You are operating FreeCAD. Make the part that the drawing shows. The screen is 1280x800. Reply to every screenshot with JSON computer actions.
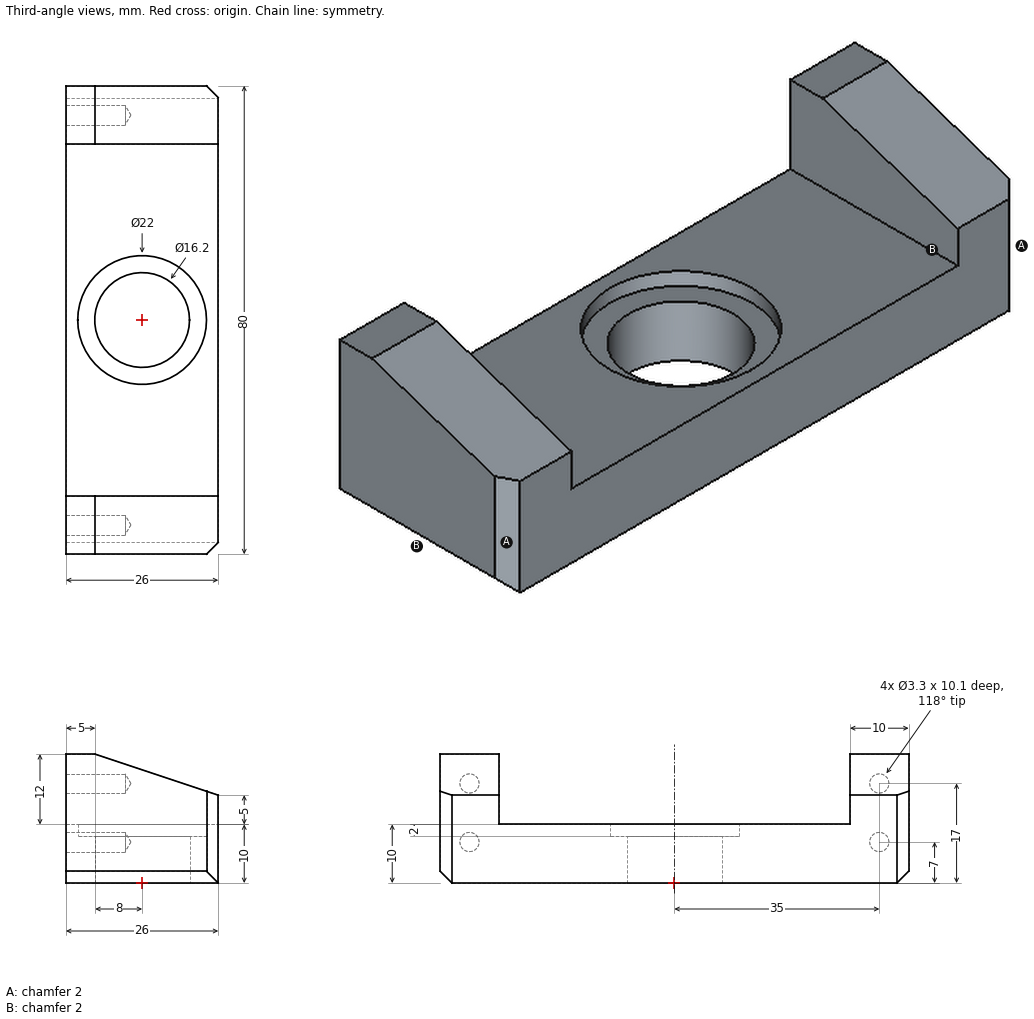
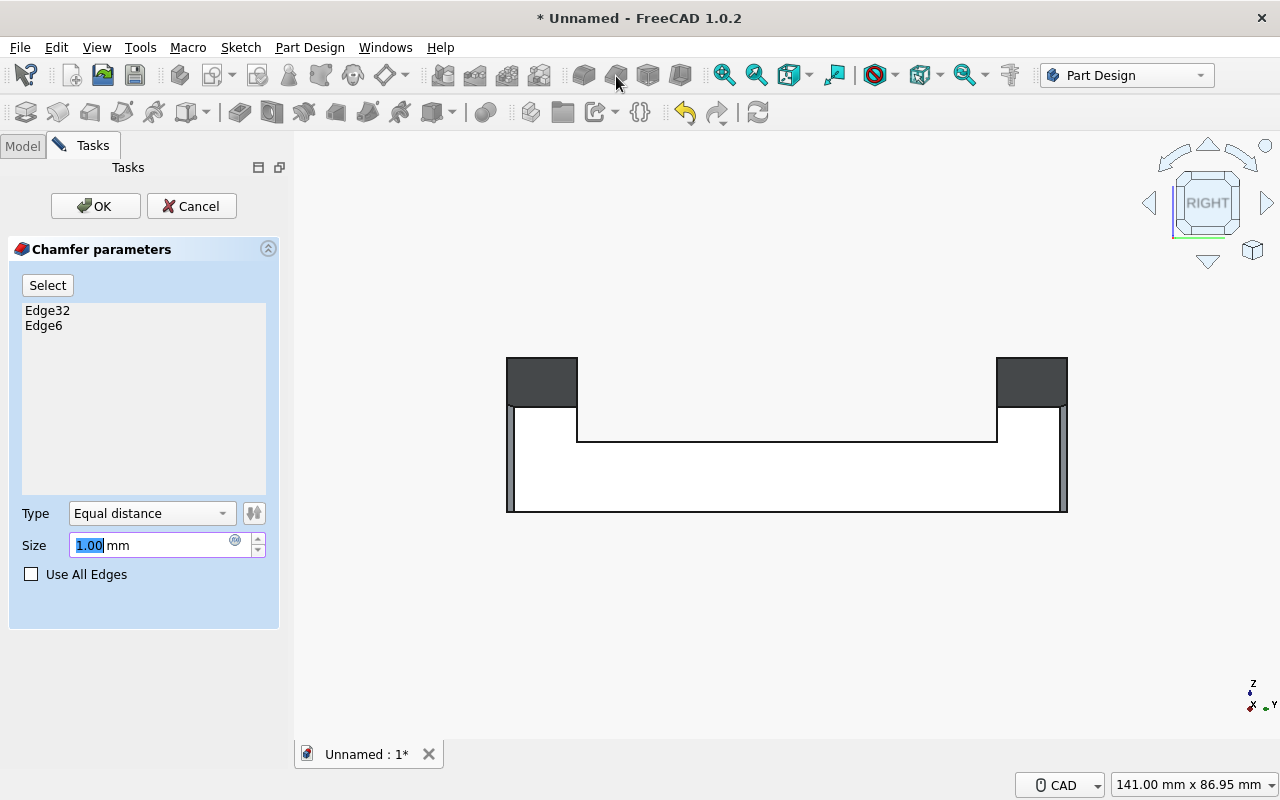
{"action": "type", "text": "2"}
{"action": "key", "text": "Tab"}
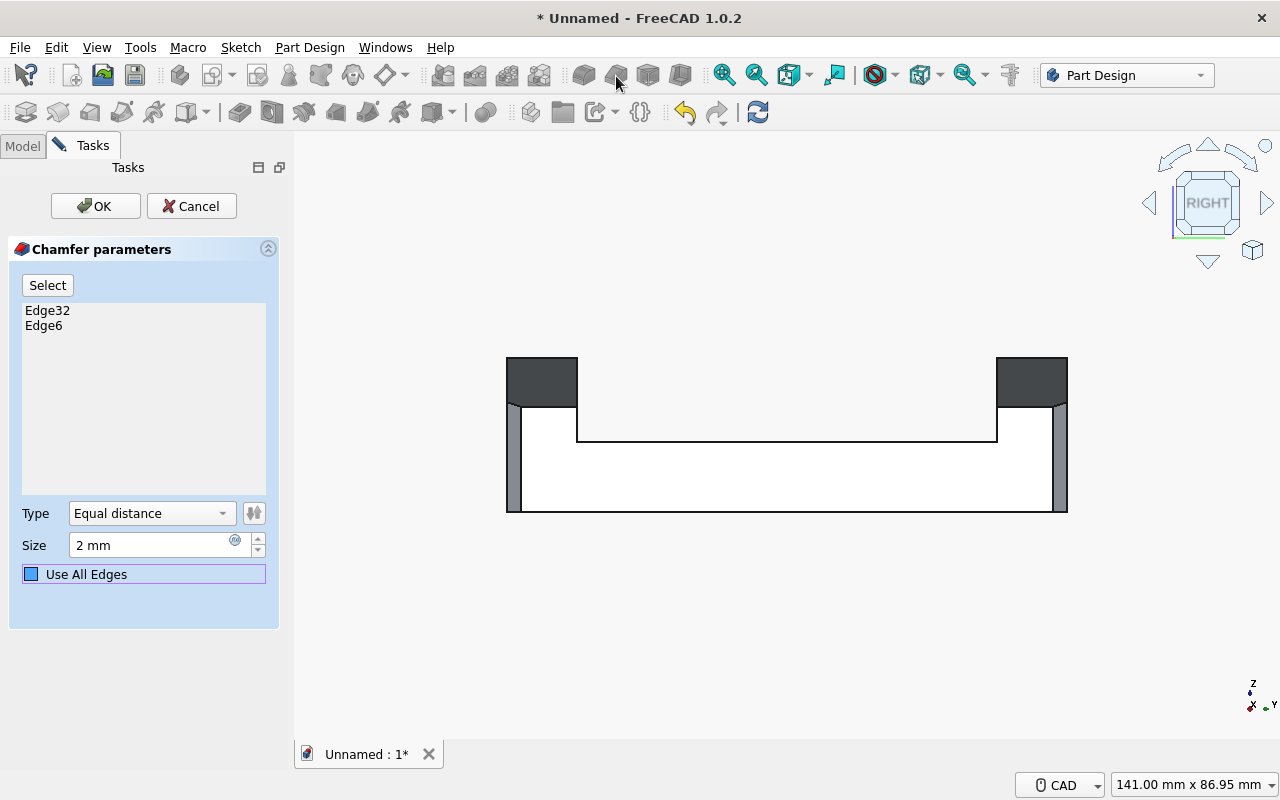
{"action": "left_click", "coordinate": [96, 206]}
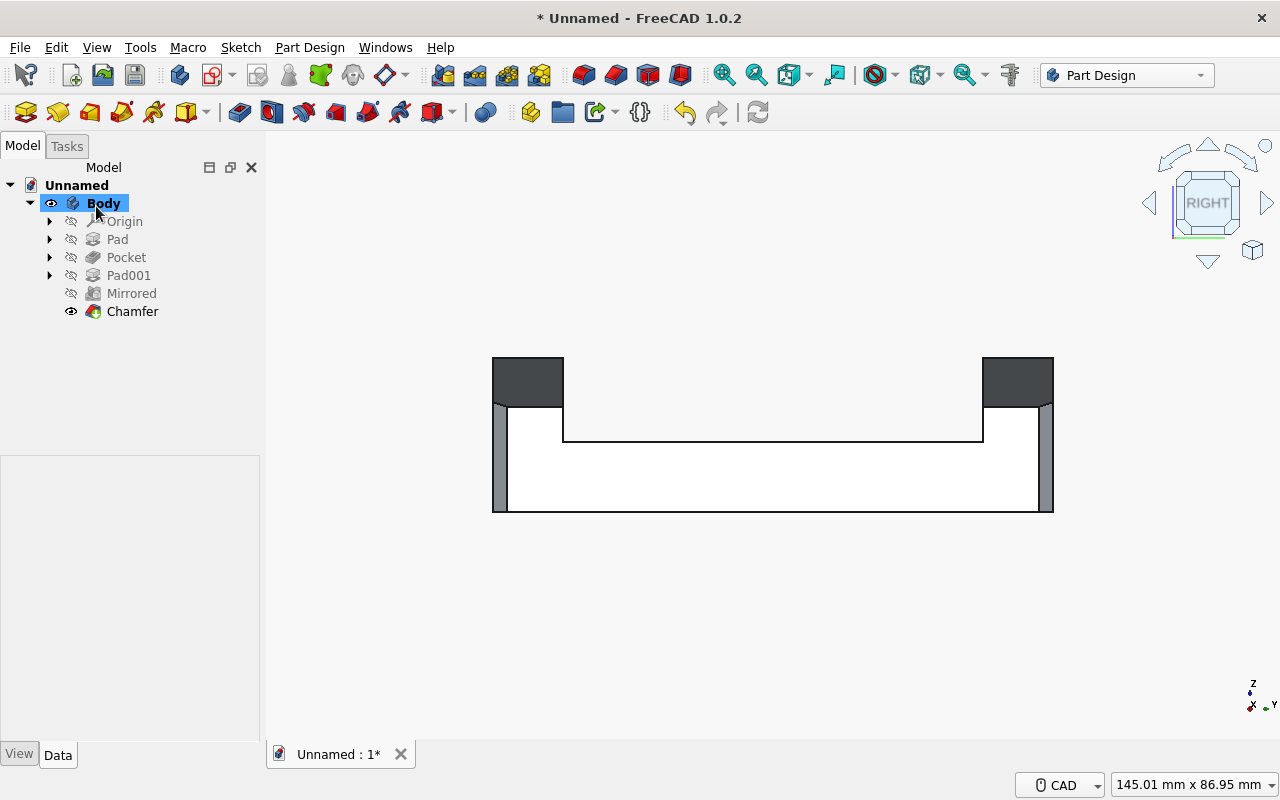
{"action": "key", "text": "0"}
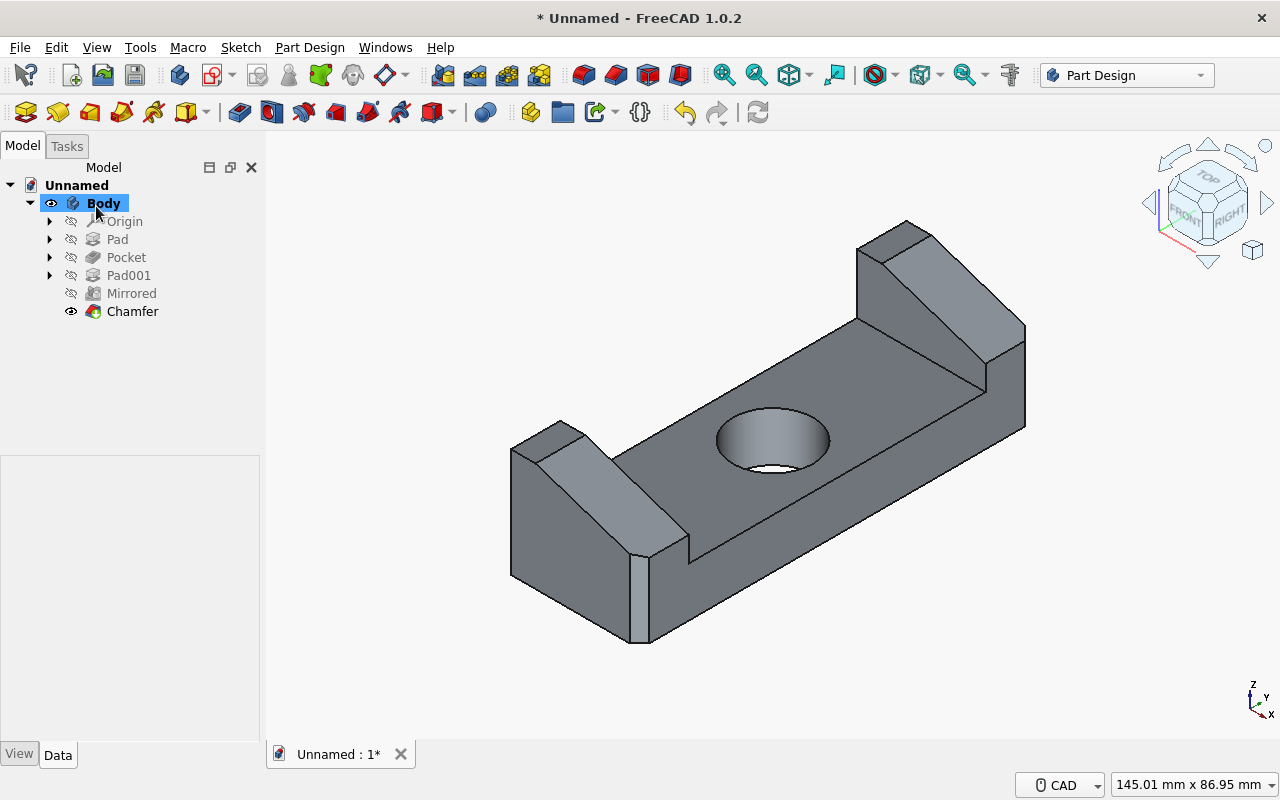
{"action": "key", "text": "2"}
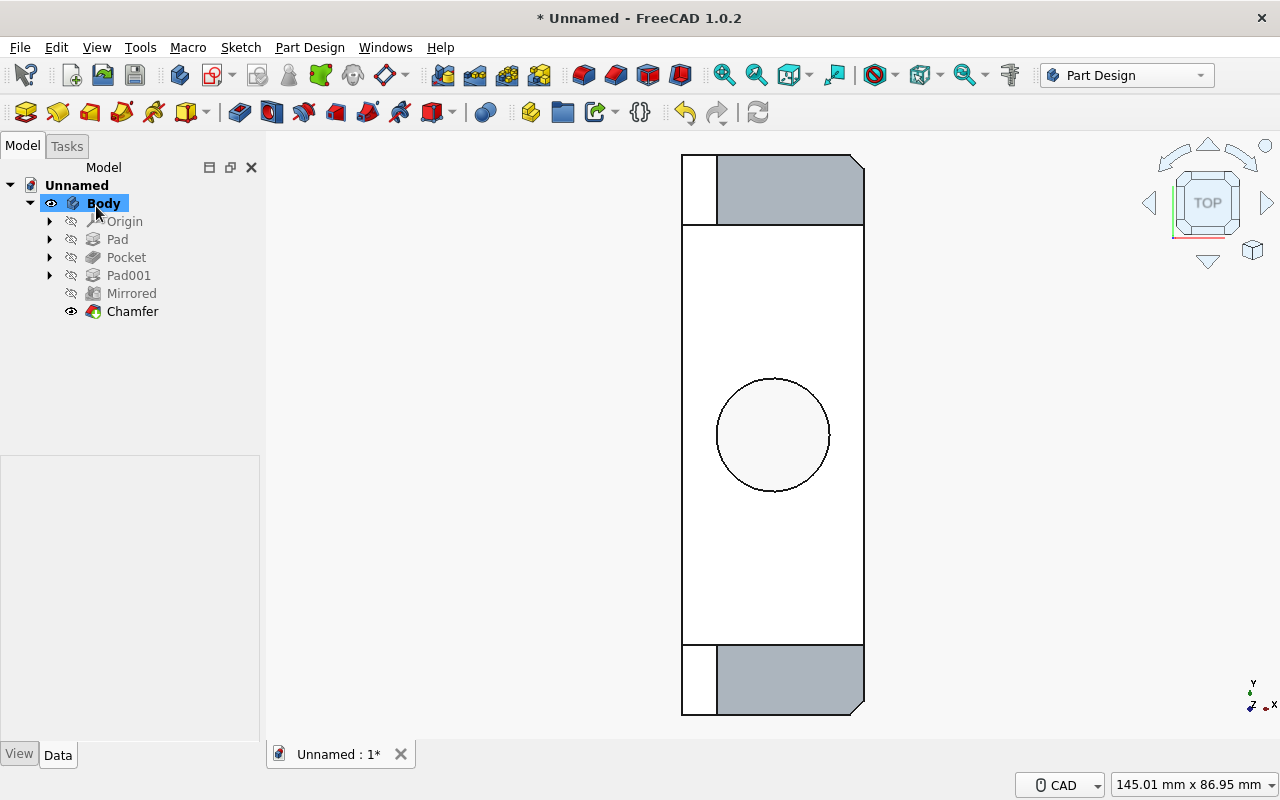
{"action": "key", "text": "1"}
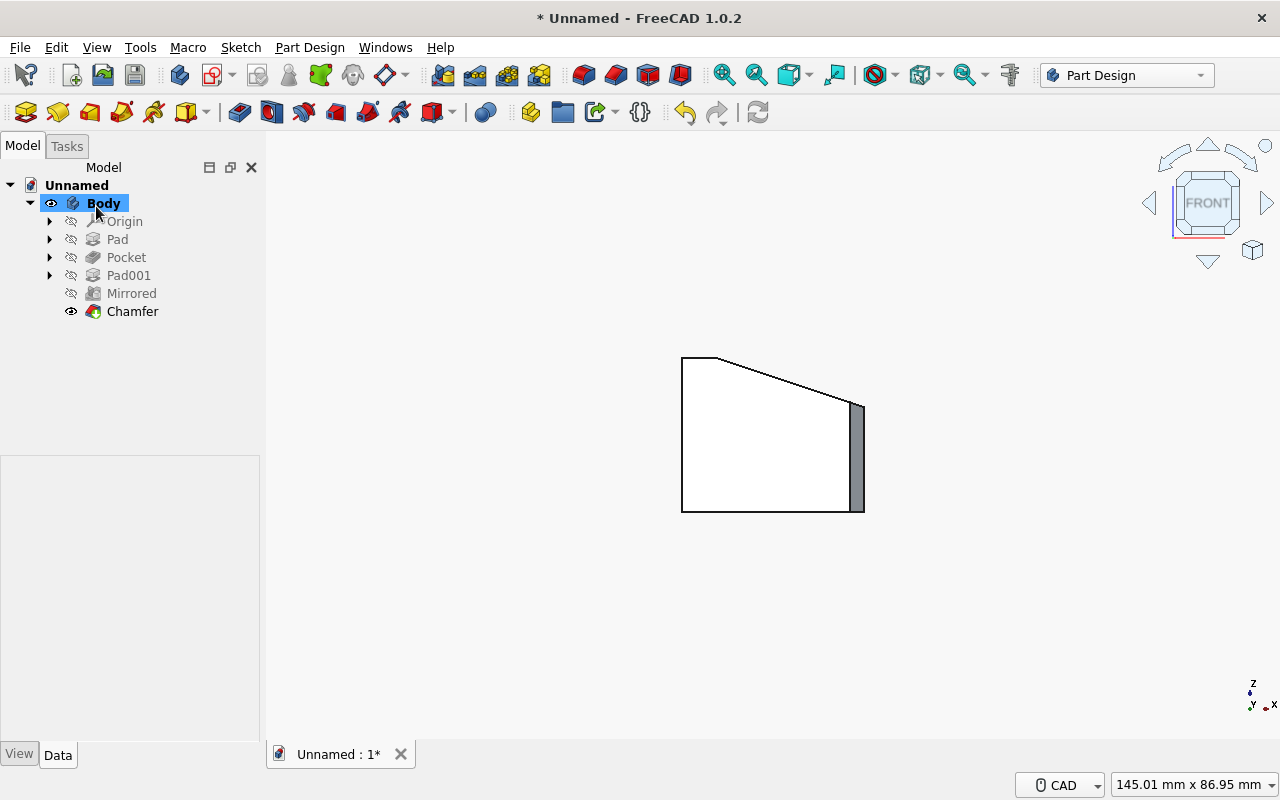
{"action": "left_click", "coordinate": [726, 76]}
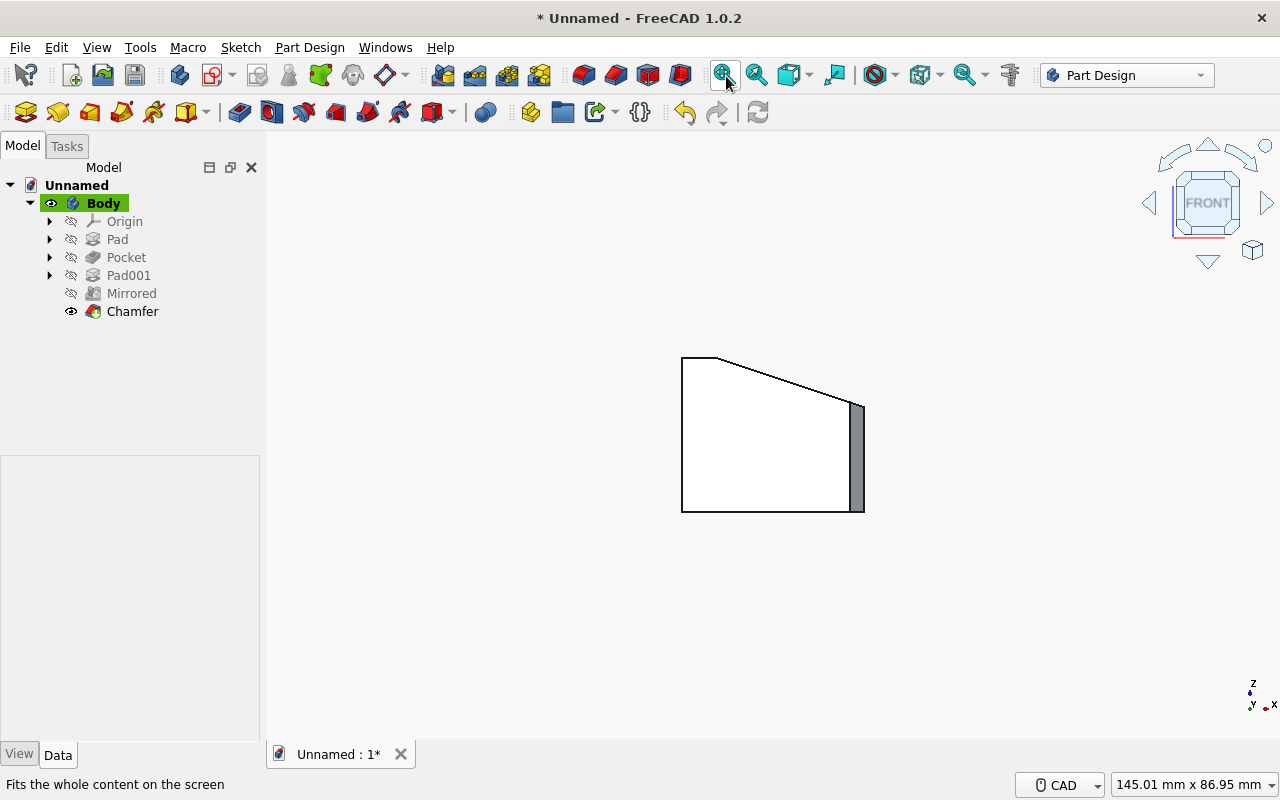
{"action": "left_click", "coordinate": [766, 511]}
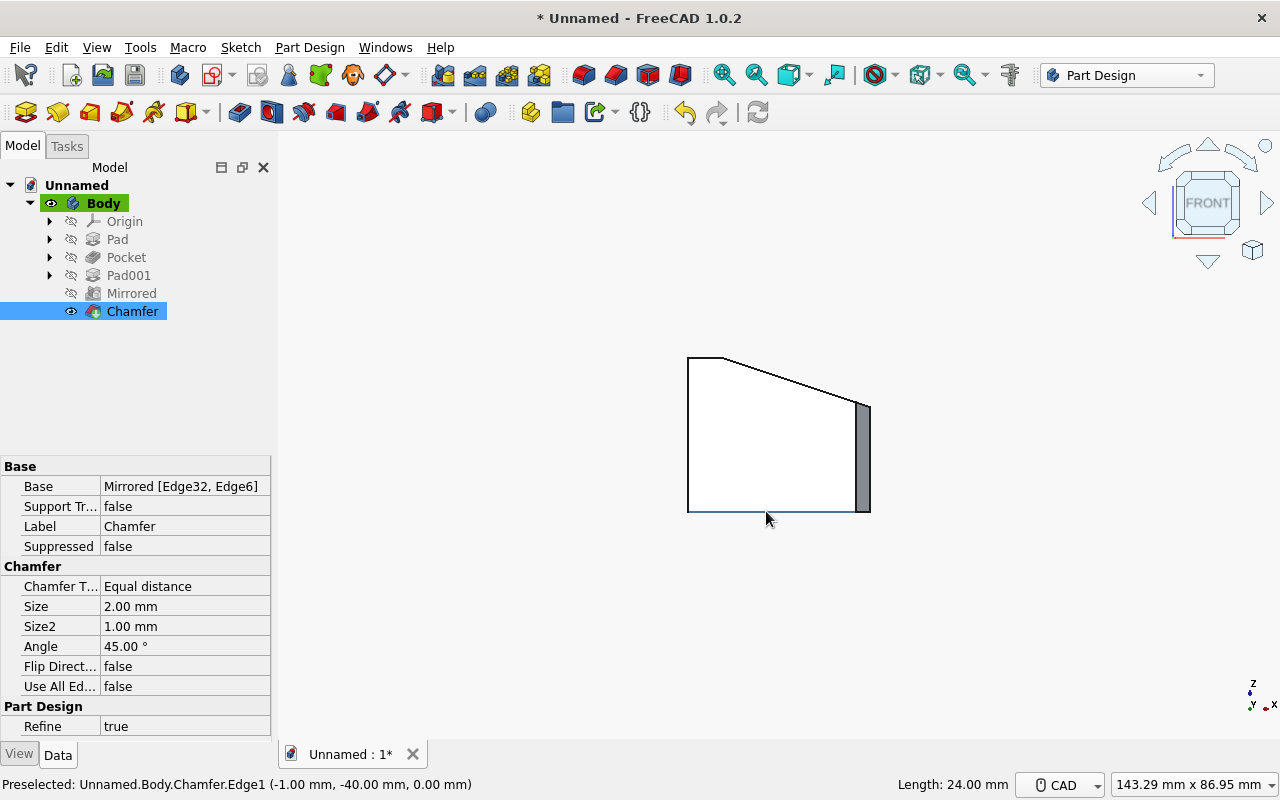
{"action": "key", "text": "3"}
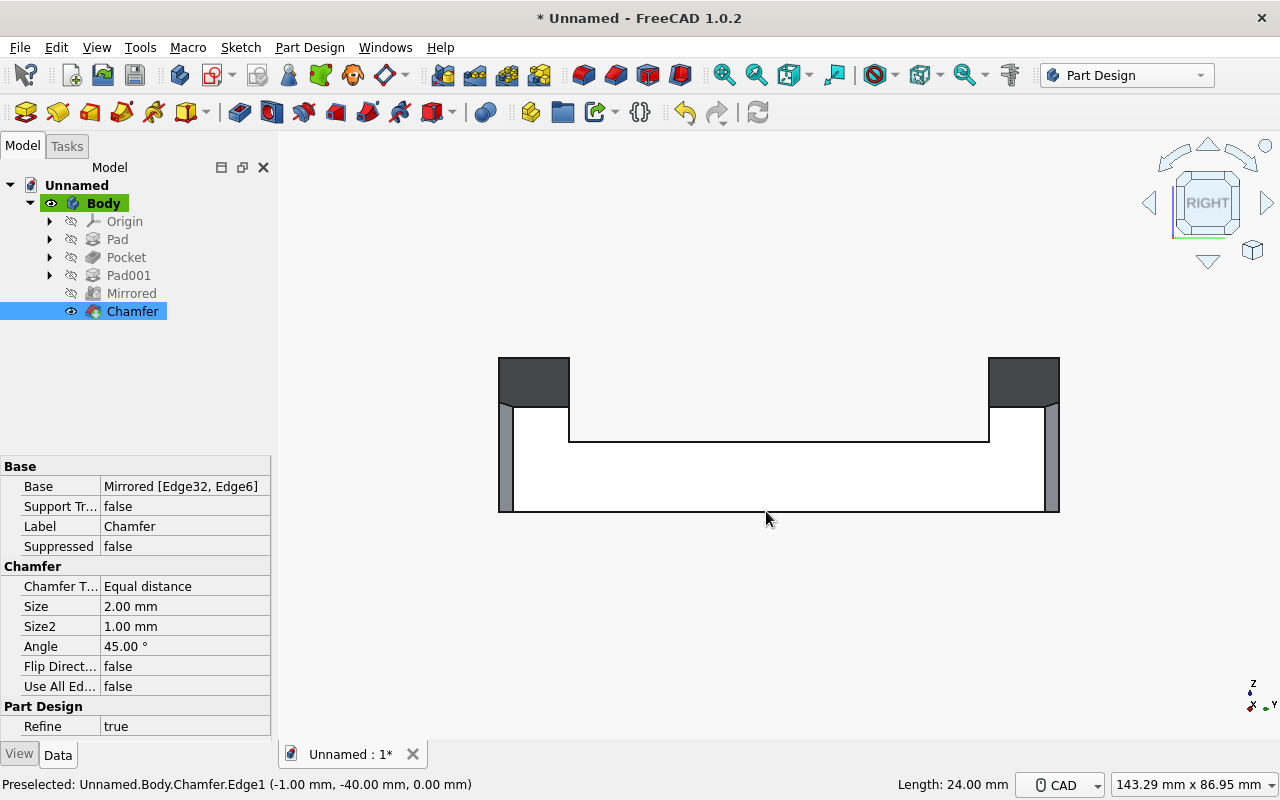
{"action": "key", "text": "5"}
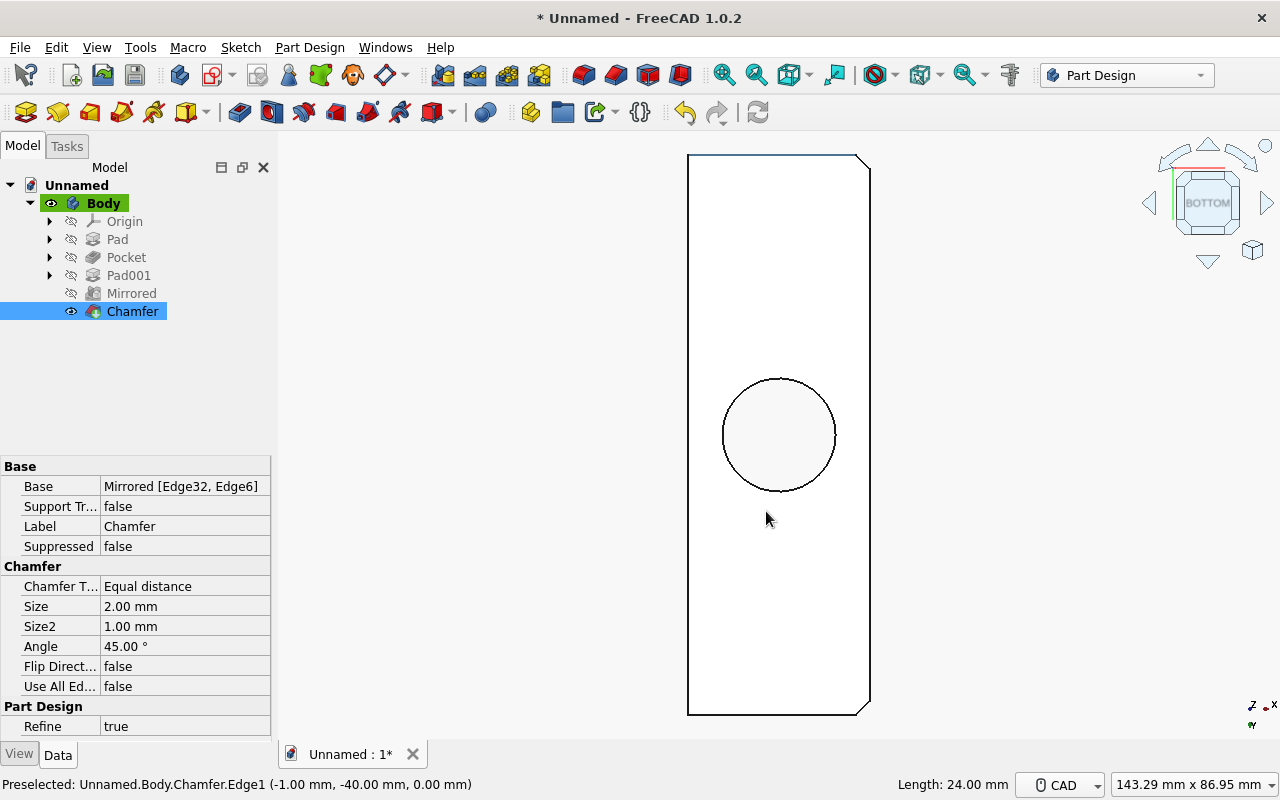
{"action": "key", "text": "4"}